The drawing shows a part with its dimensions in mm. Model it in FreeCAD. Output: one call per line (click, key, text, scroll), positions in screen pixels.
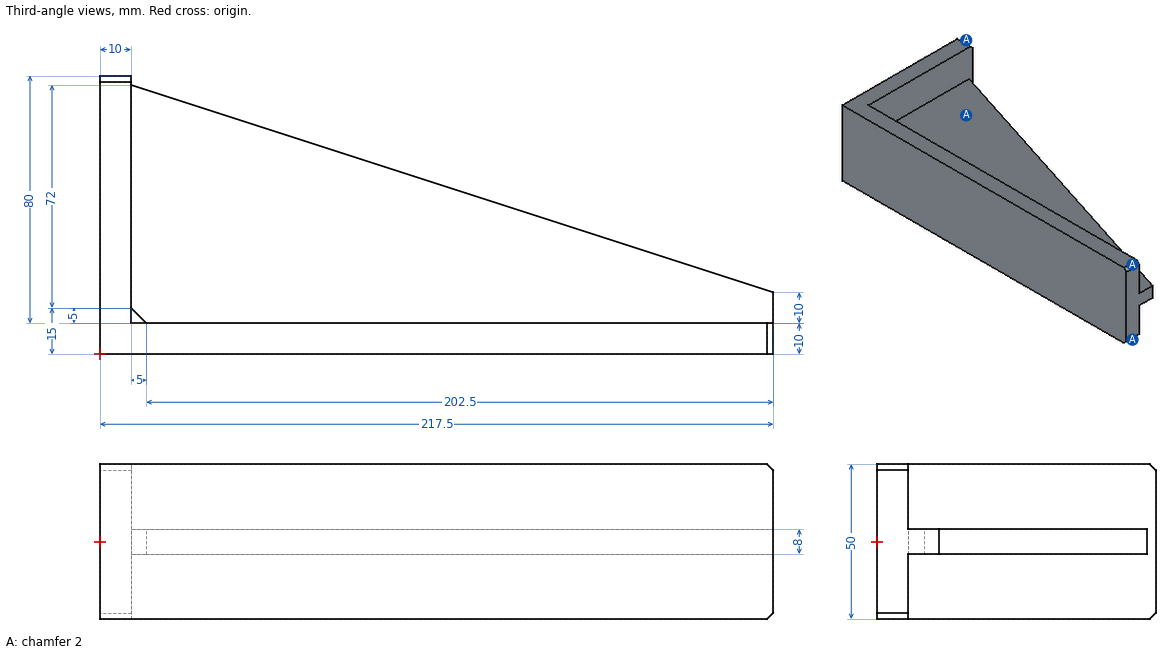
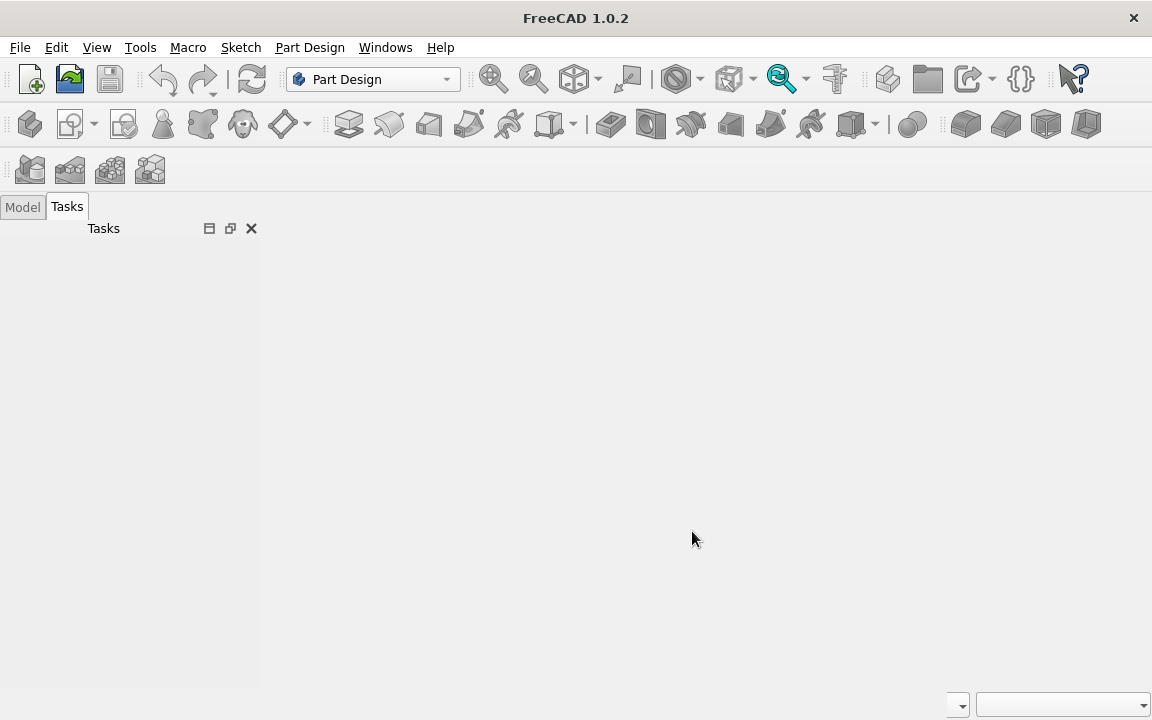
click(30, 80)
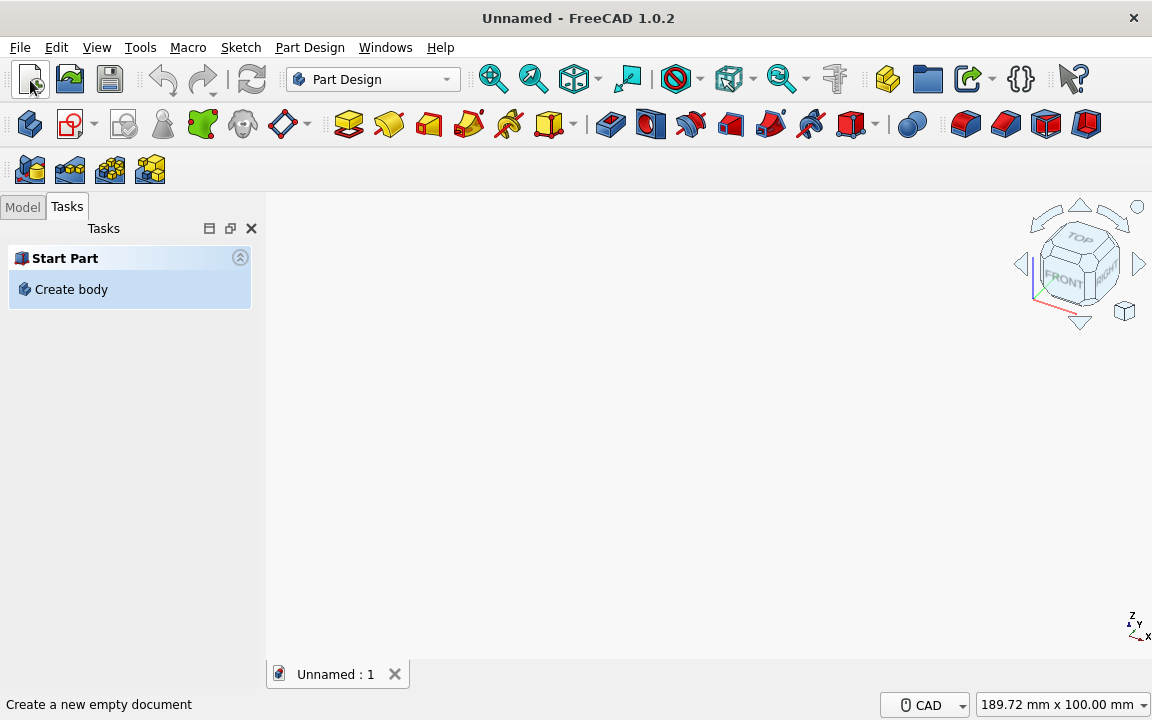
click(70, 124)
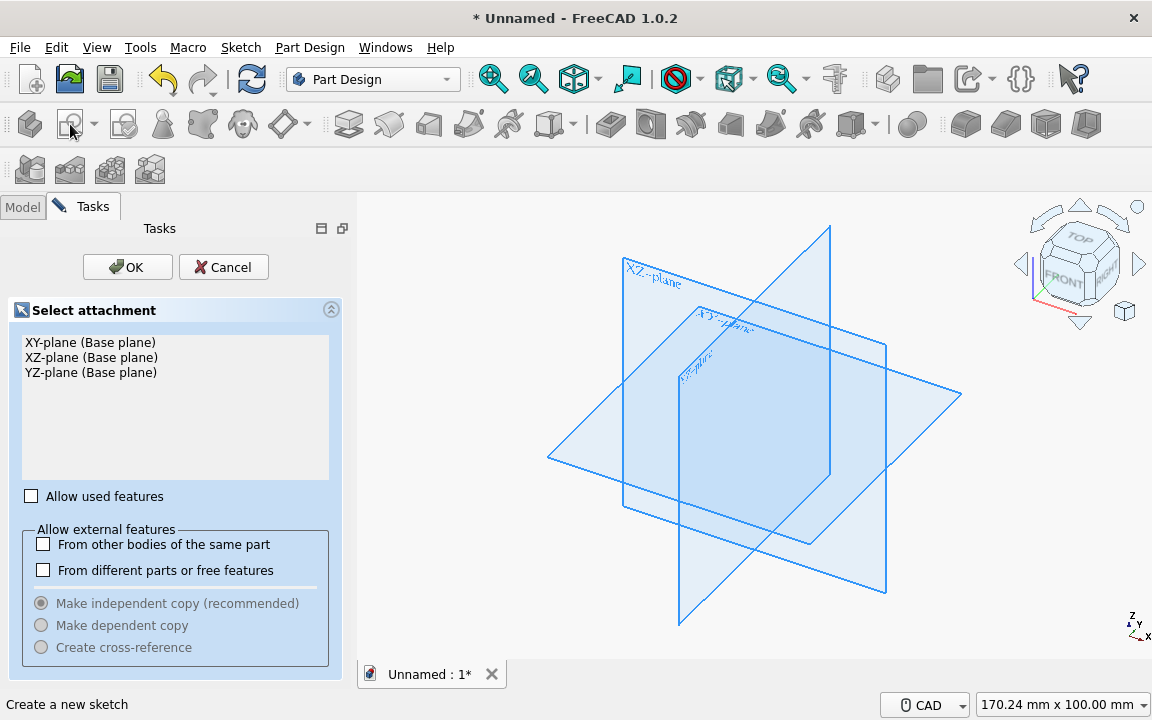
click(82, 342)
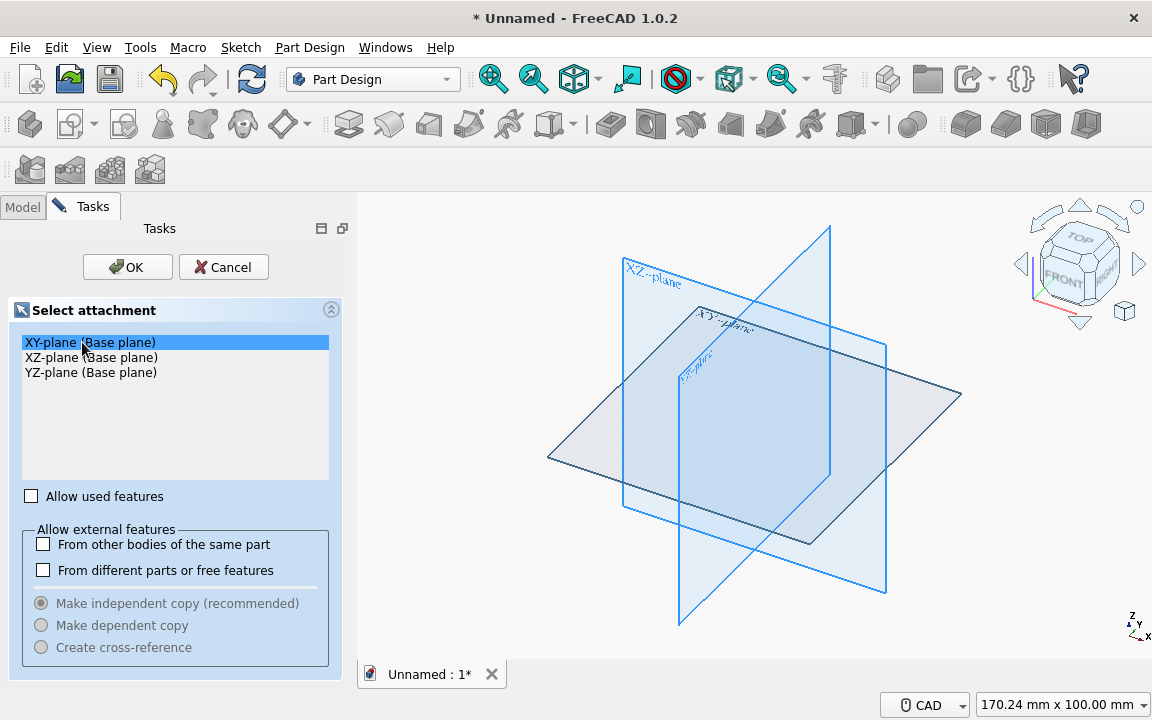
click(128, 267)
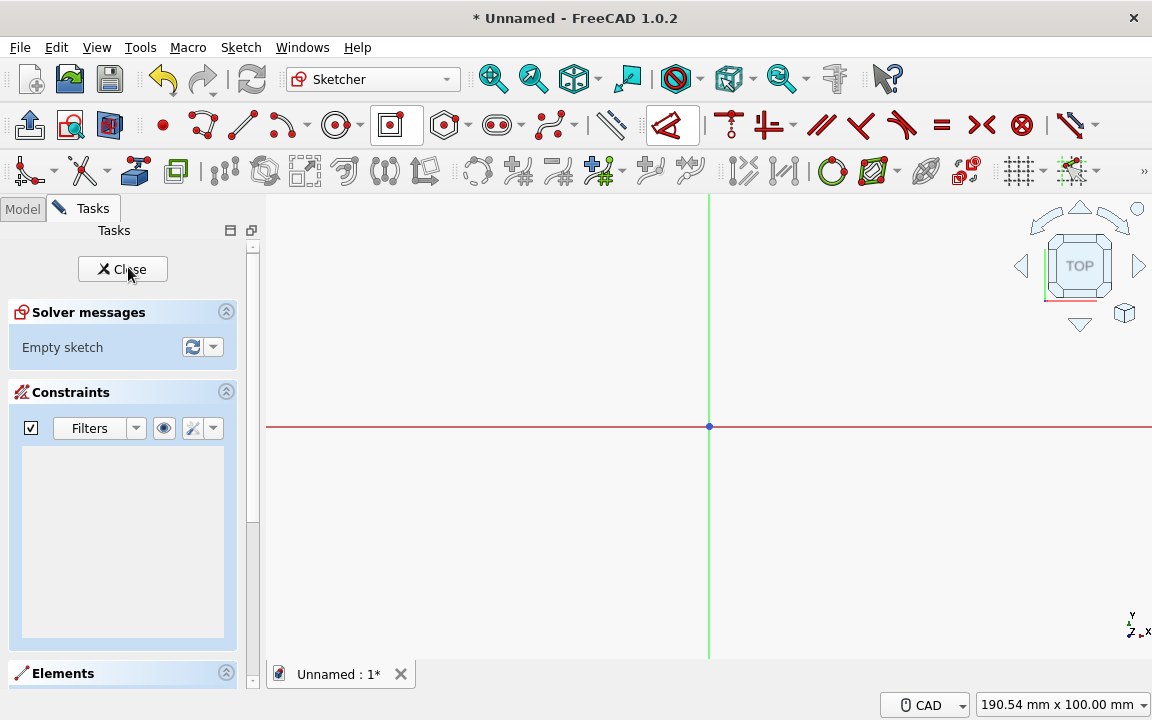
scroll(294, 597, down, 4)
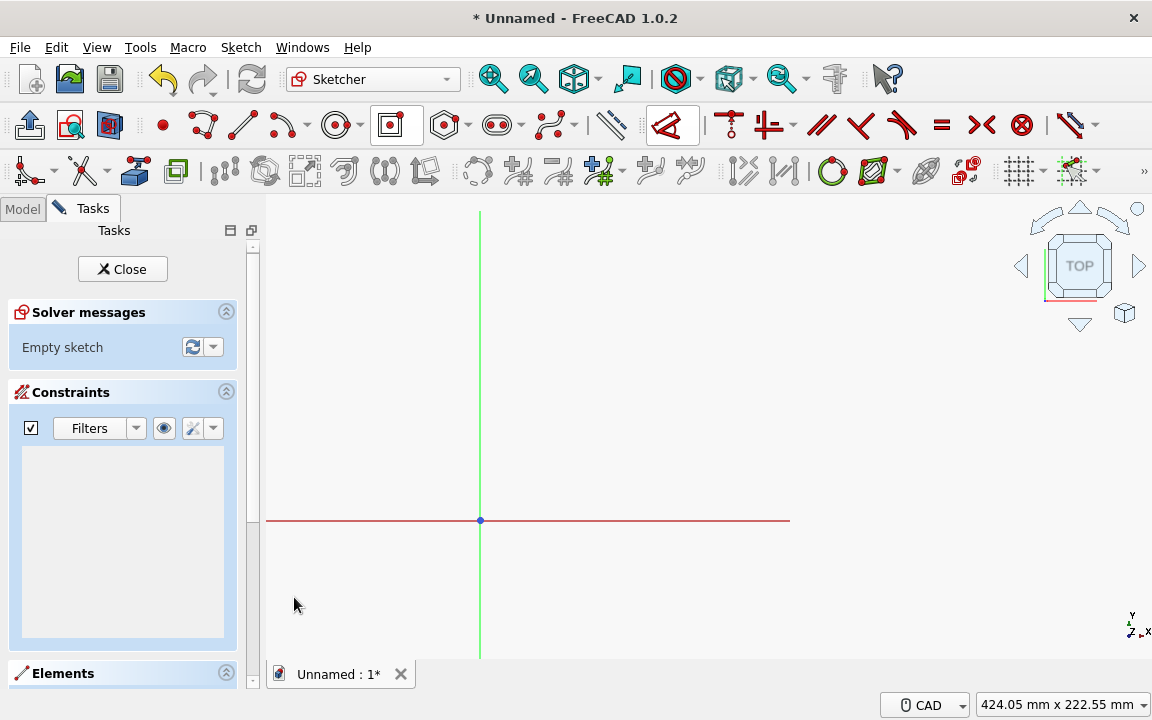
click(204, 126)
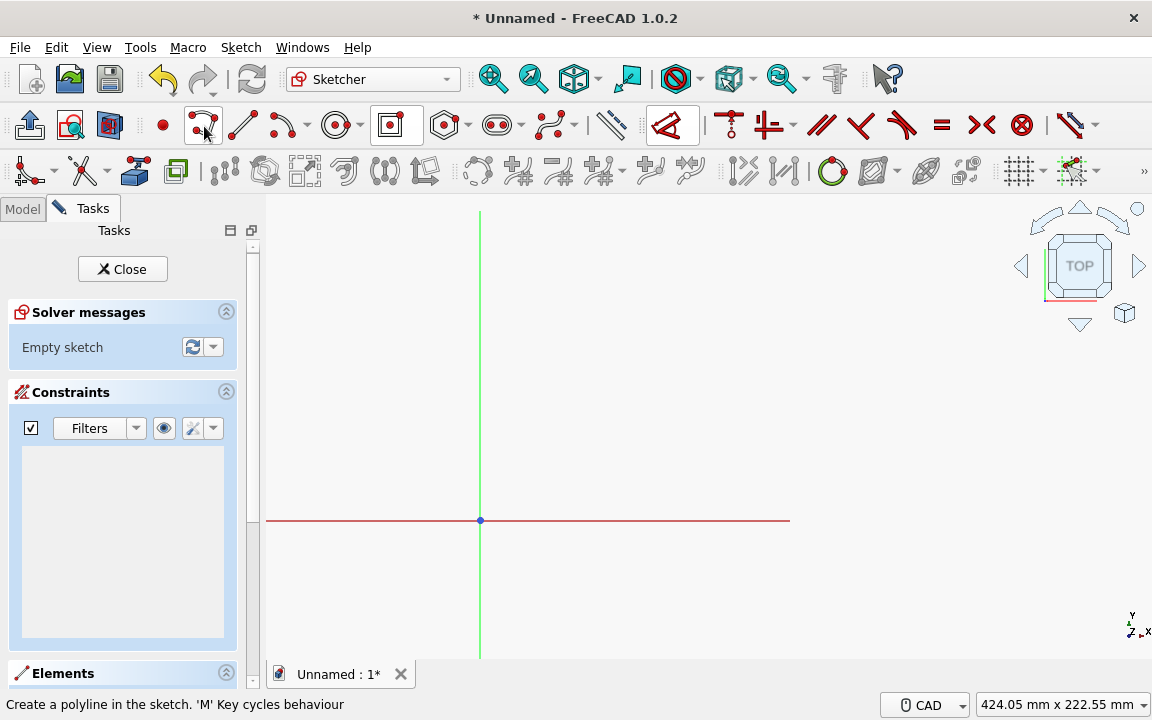
click(480, 521)
click(935, 512)
click(935, 500)
click(501, 500)
click(501, 333)
click(489, 333)
click(480, 521)
key(Escape)
key(Escape)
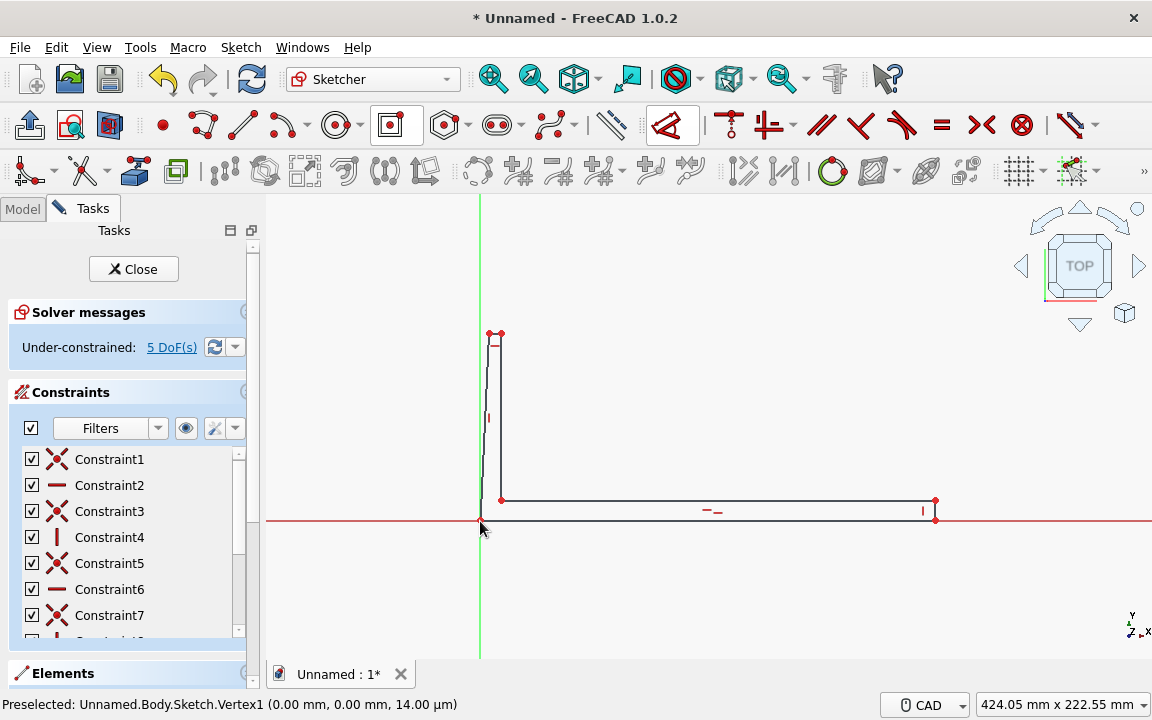
click(483, 465)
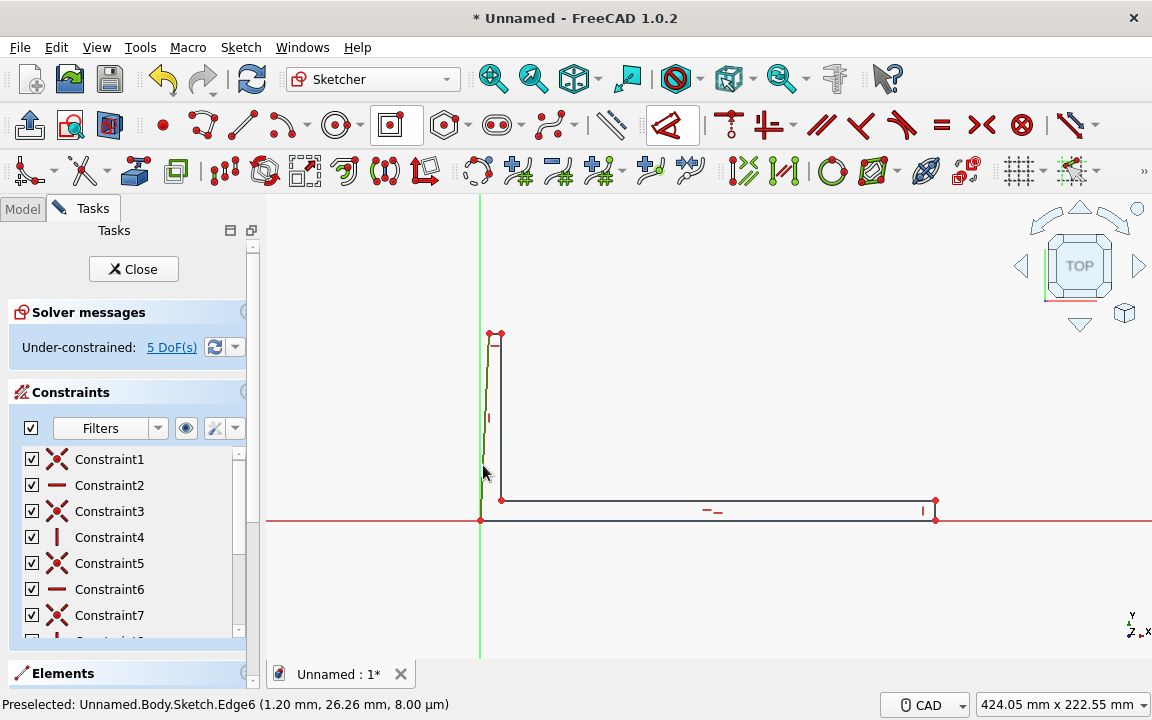
click(796, 126)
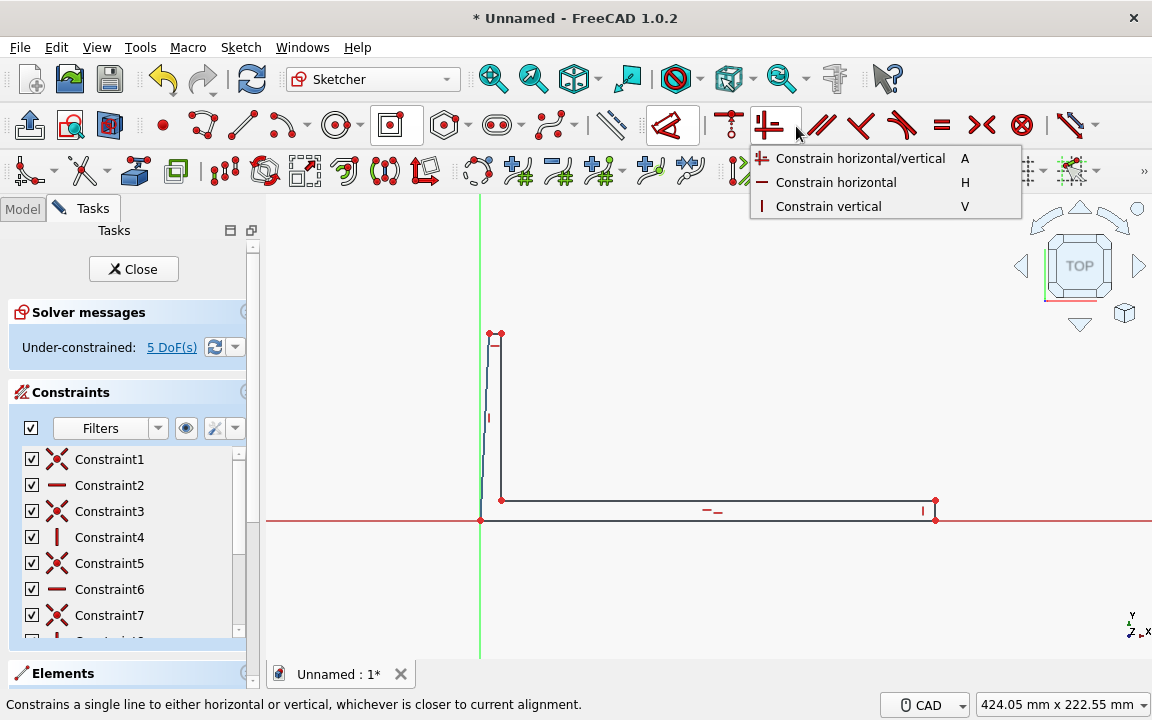
click(886, 206)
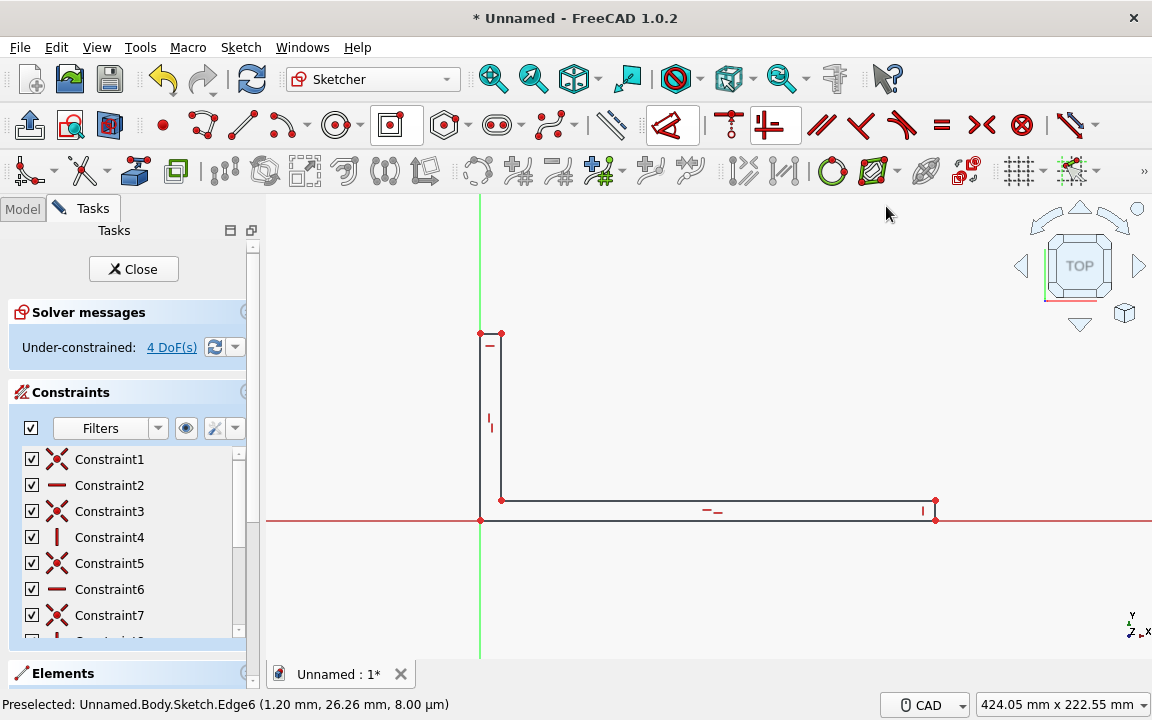
click(666, 126)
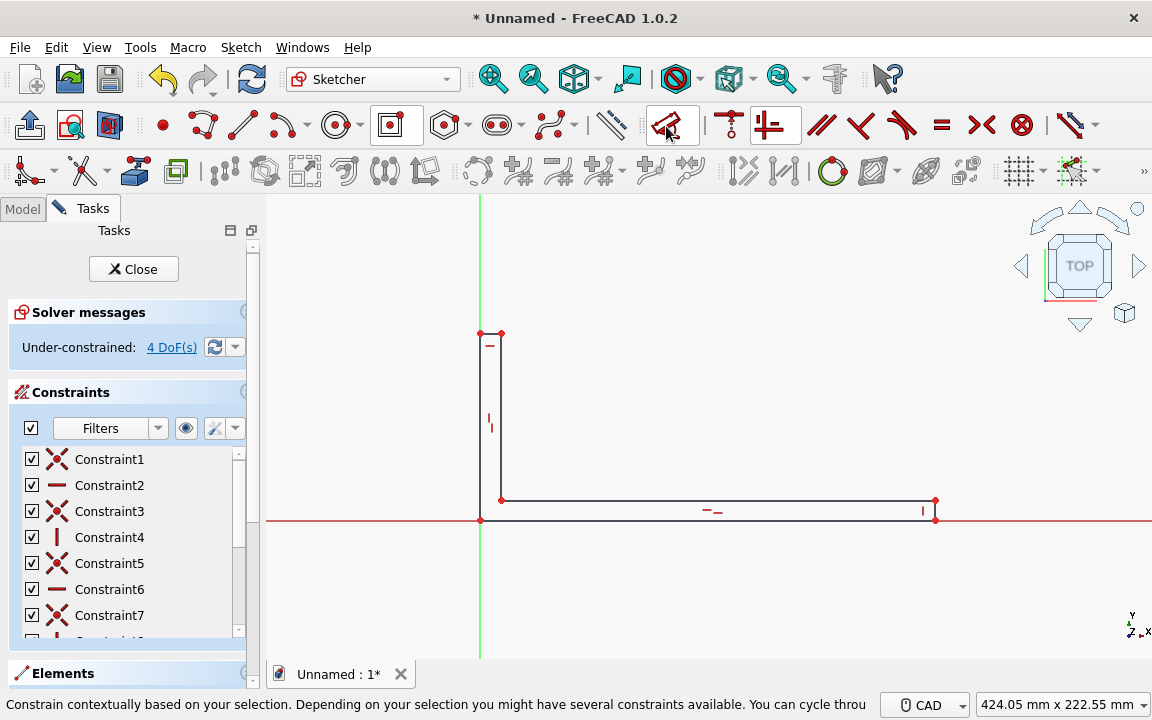
scroll(935, 511, up, 4)